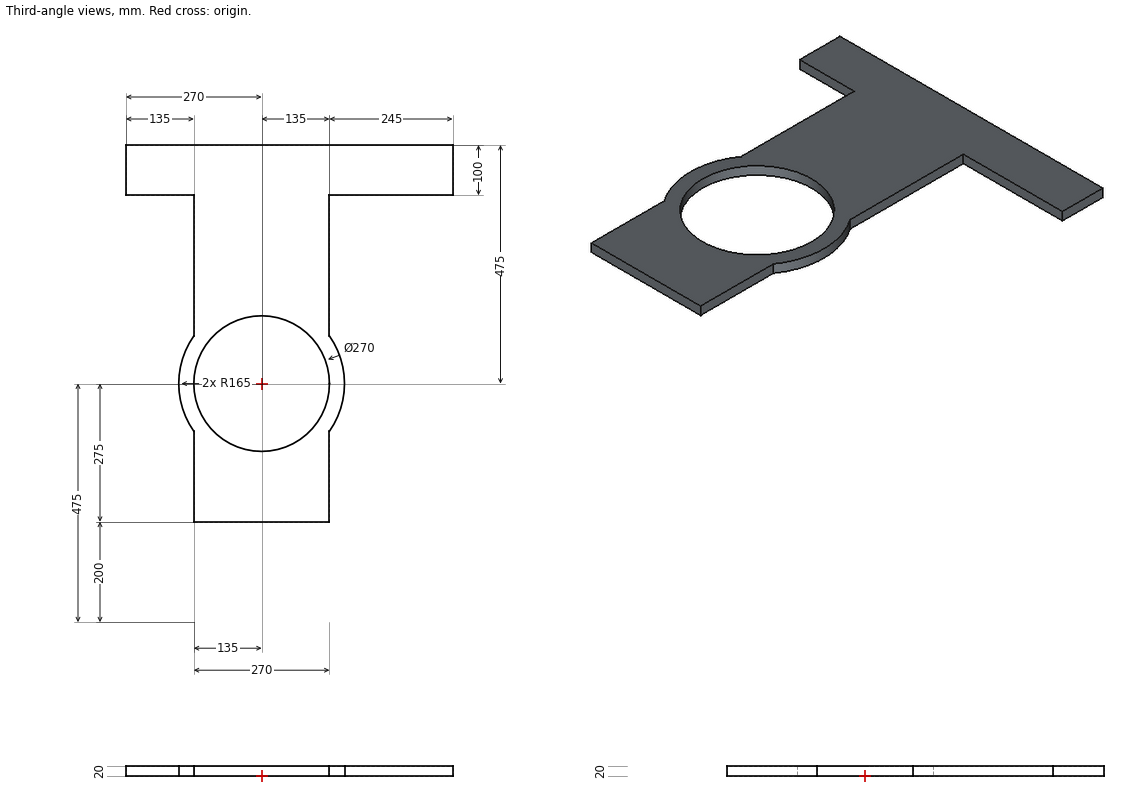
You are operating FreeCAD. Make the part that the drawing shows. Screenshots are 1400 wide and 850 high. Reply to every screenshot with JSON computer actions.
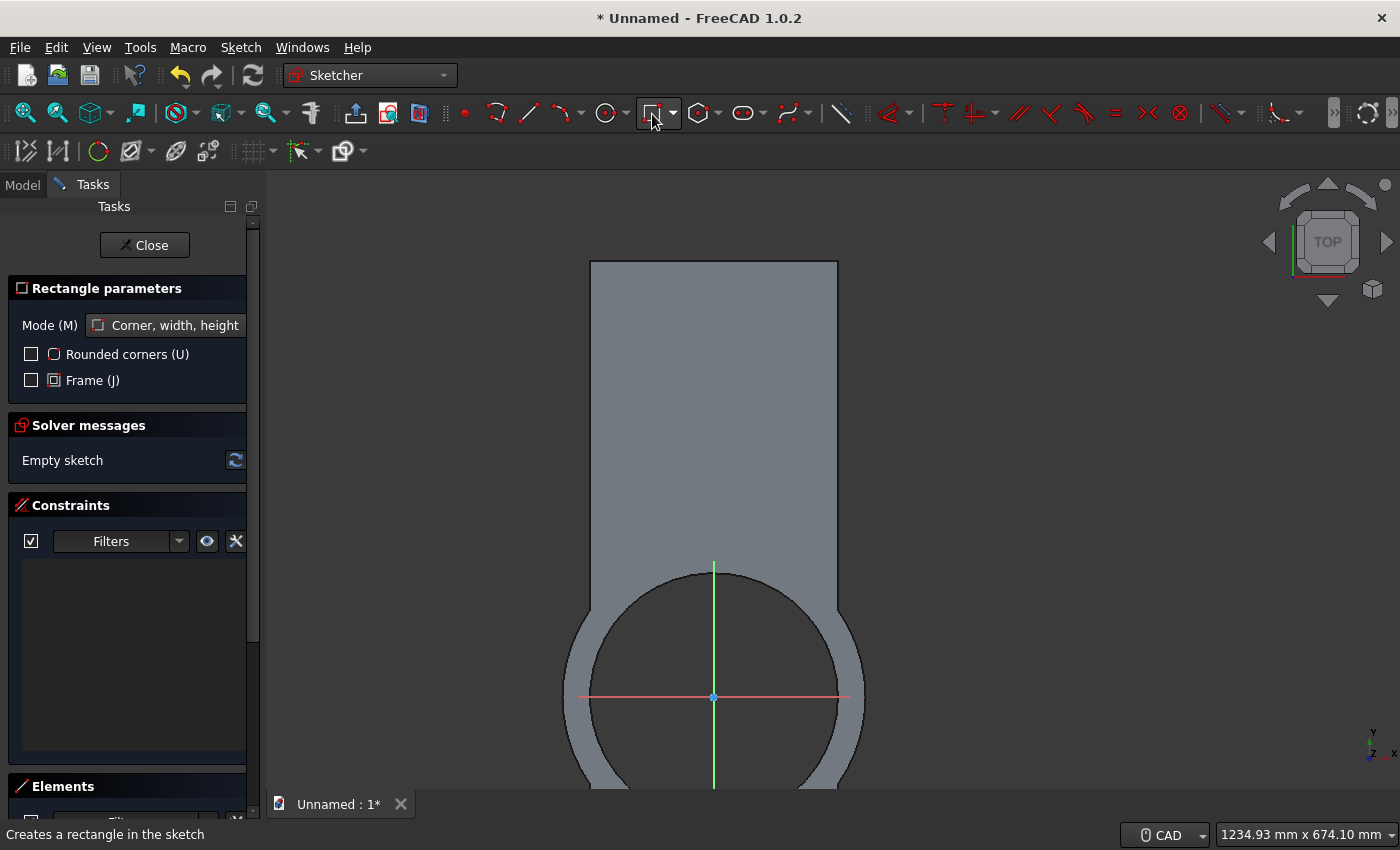
{"action": "left_click", "coordinate": [838, 261]}
{"action": "left_click", "coordinate": [1063, 353]}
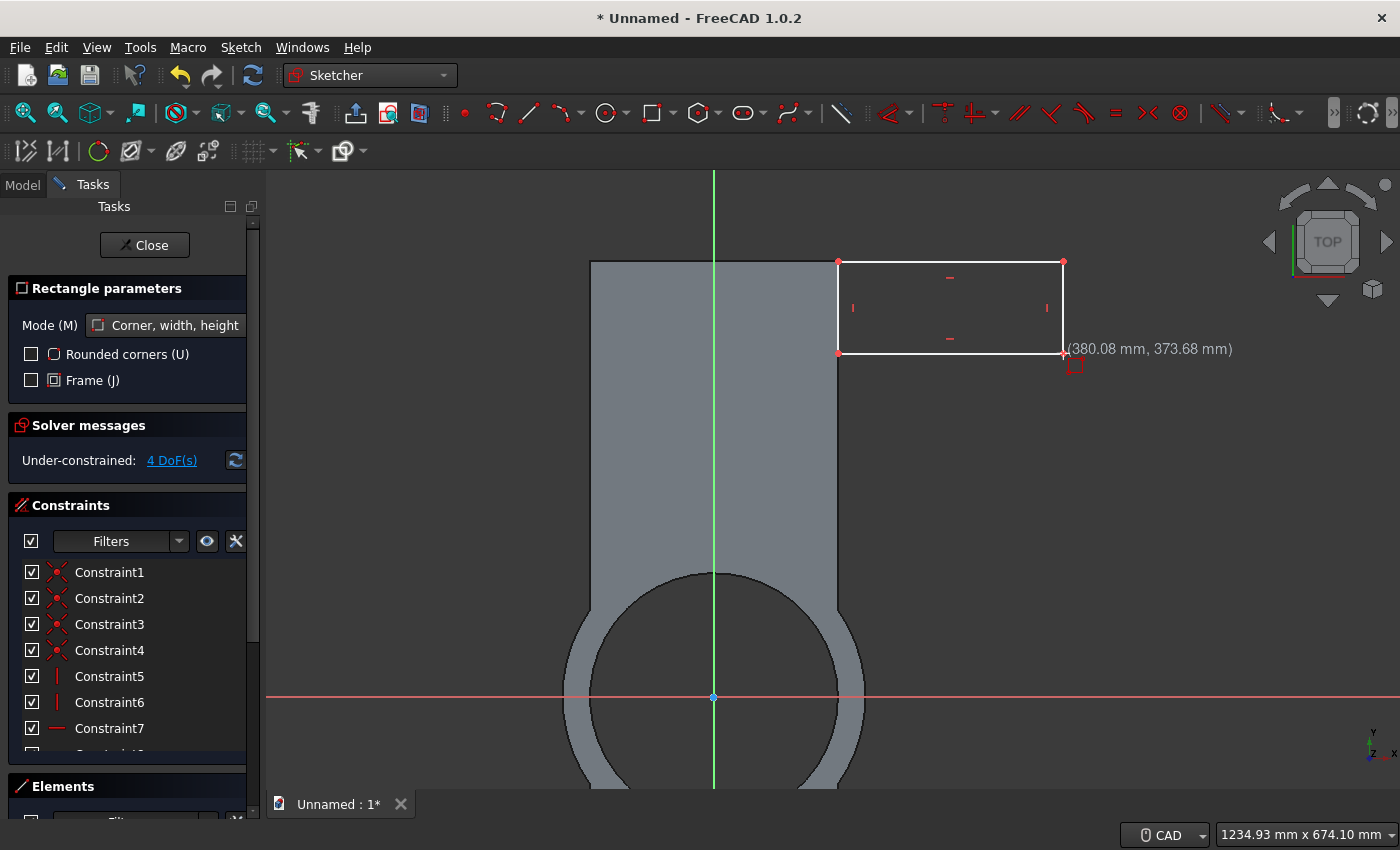
{"action": "left_click", "coordinate": [466, 261]}
{"action": "left_click", "coordinate": [590, 353]}
{"action": "key", "text": "Escape"}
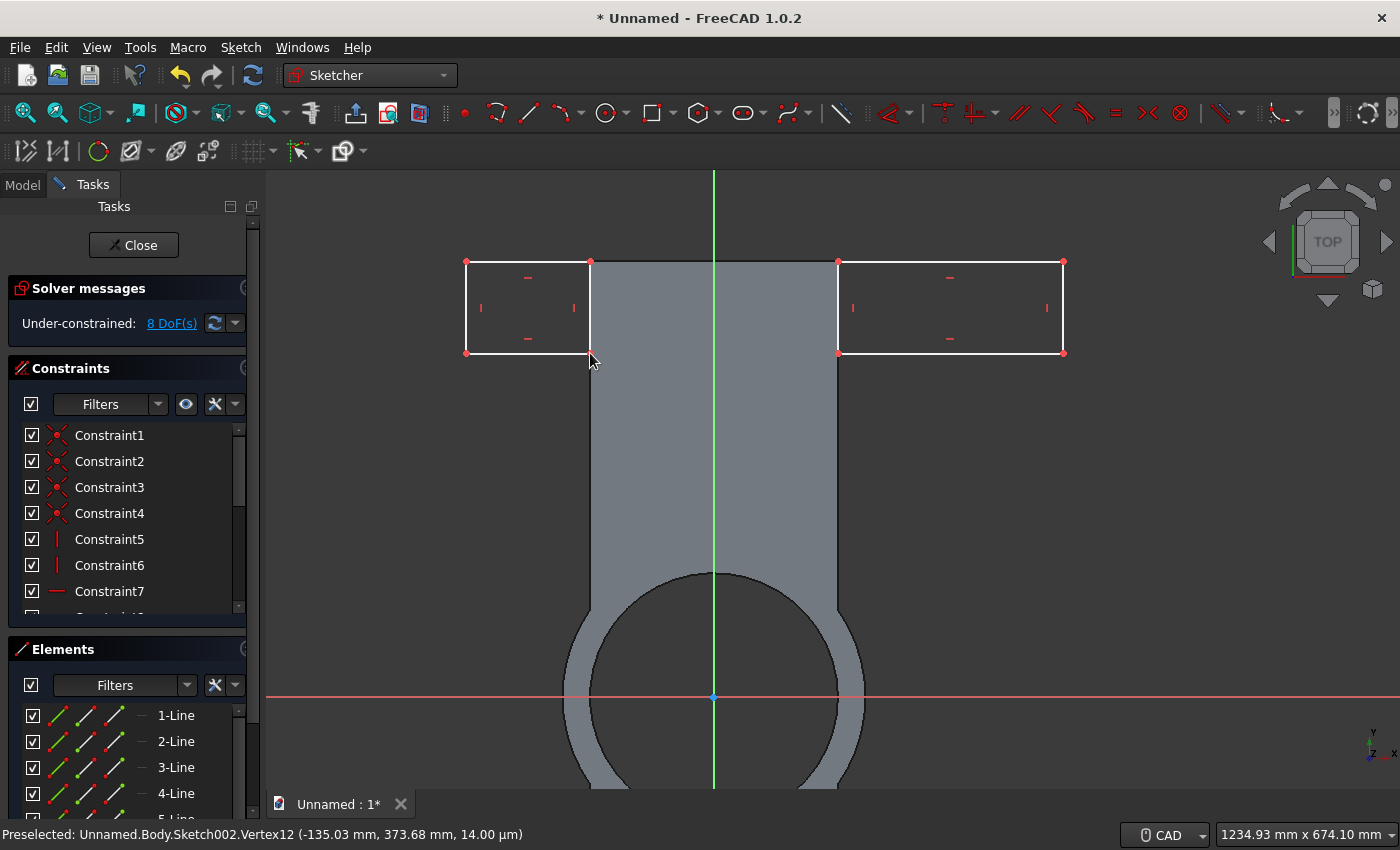
{"action": "left_click", "coordinate": [888, 114]}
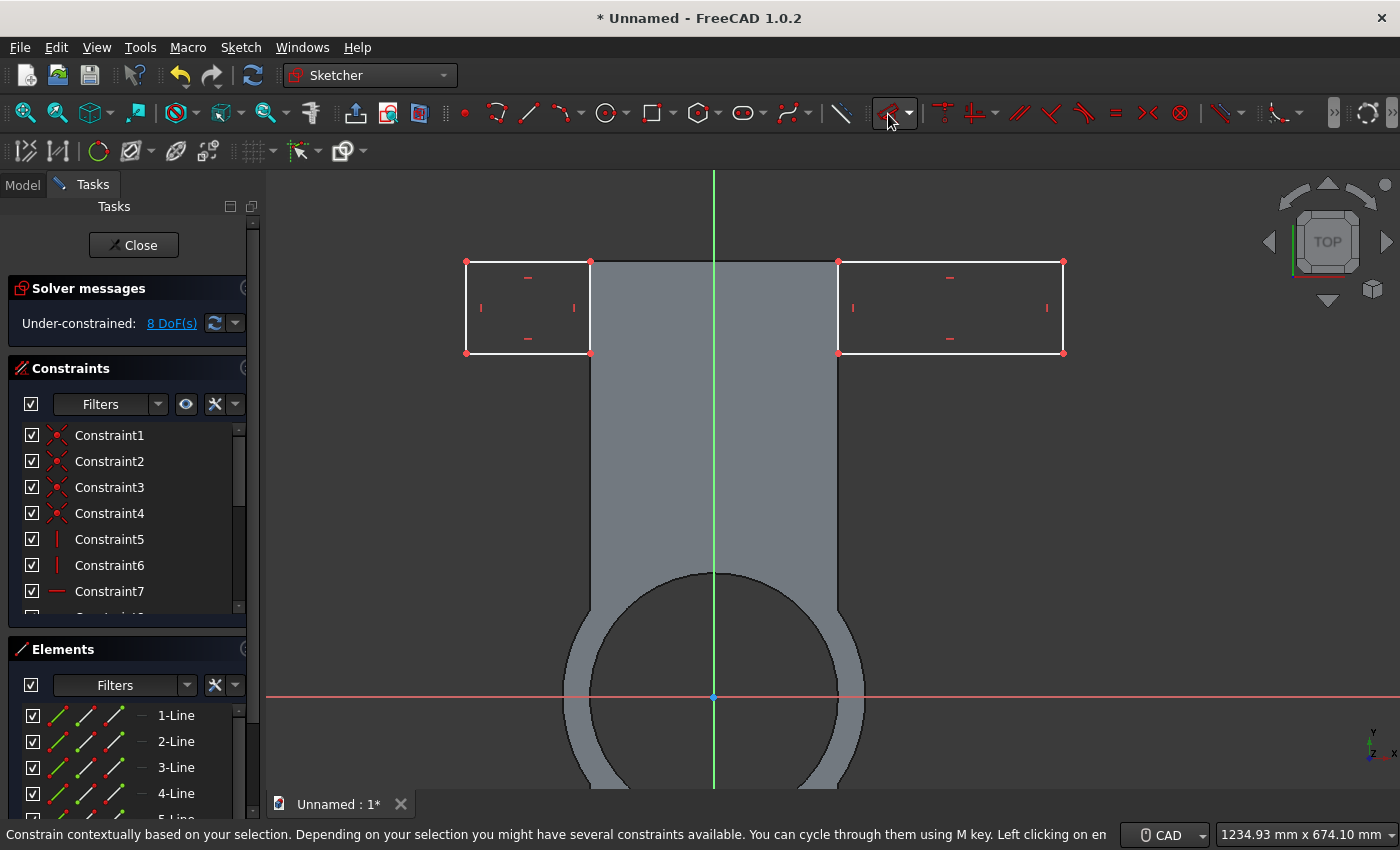
{"action": "left_click", "coordinate": [838, 290]}
{"action": "left_click", "coordinate": [872, 308]}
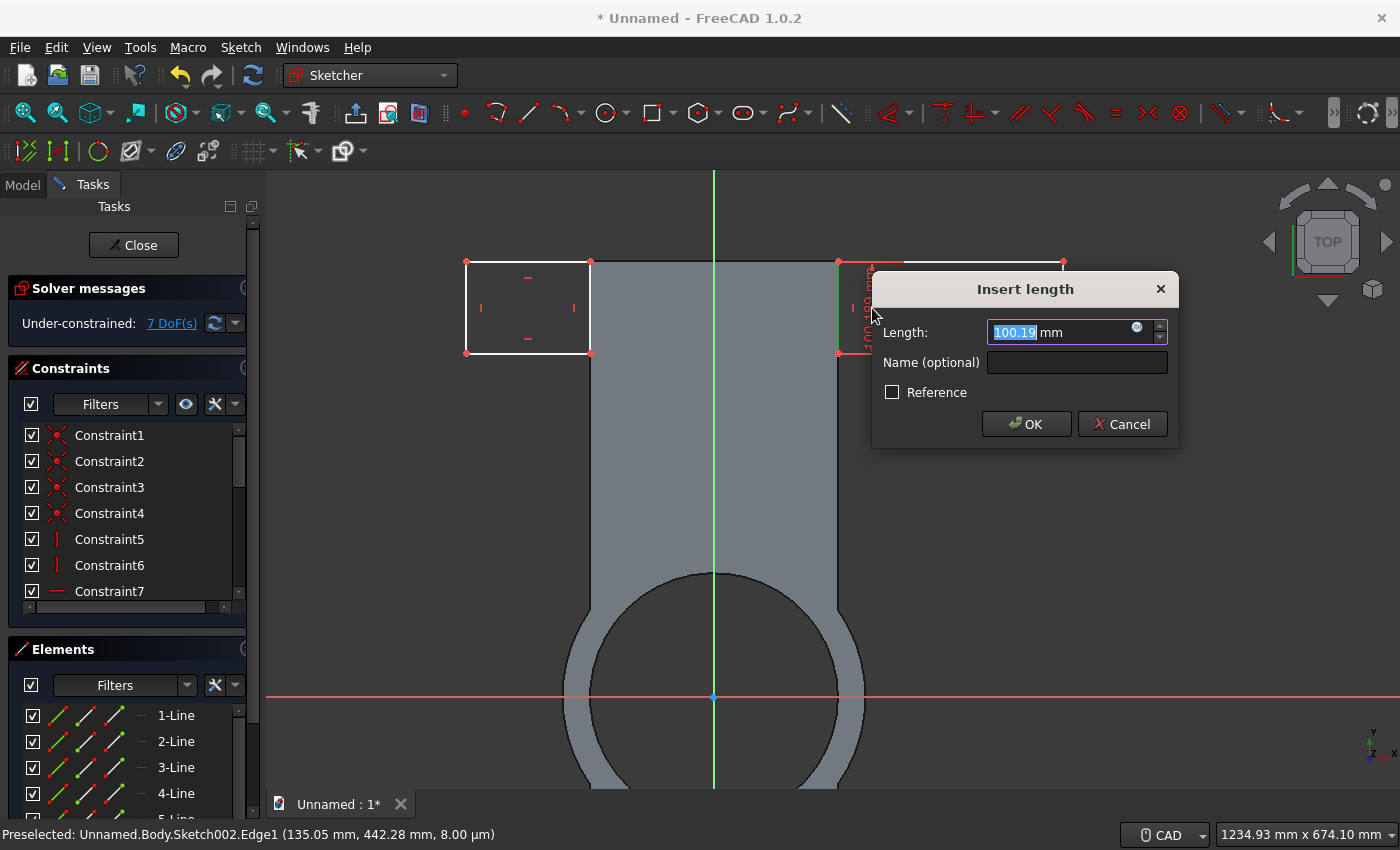
{"action": "type", "text": "100"}
{"action": "key", "text": "Return"}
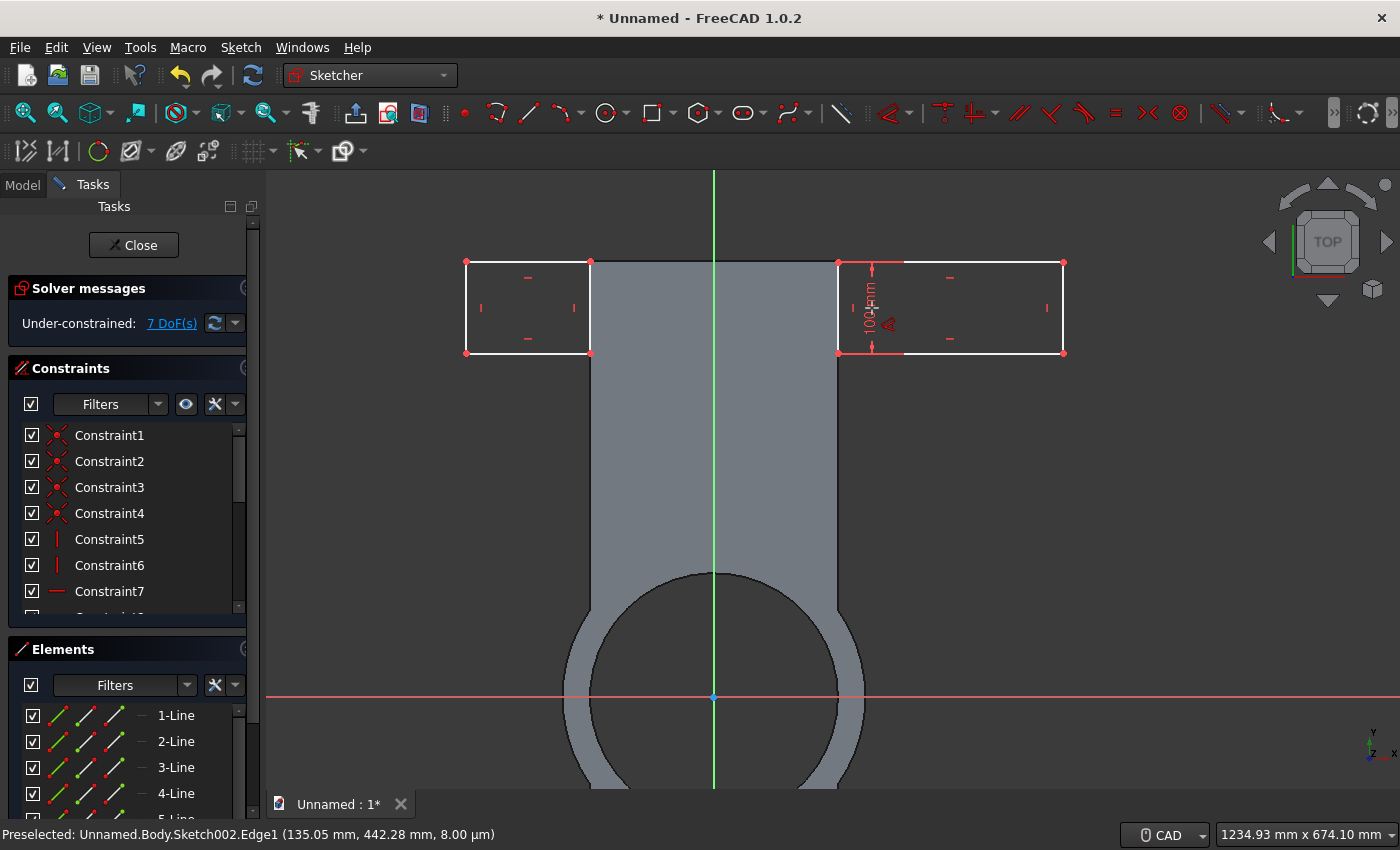
{"action": "left_click", "coordinate": [906, 354]}
{"action": "left_click", "coordinate": [950, 320]}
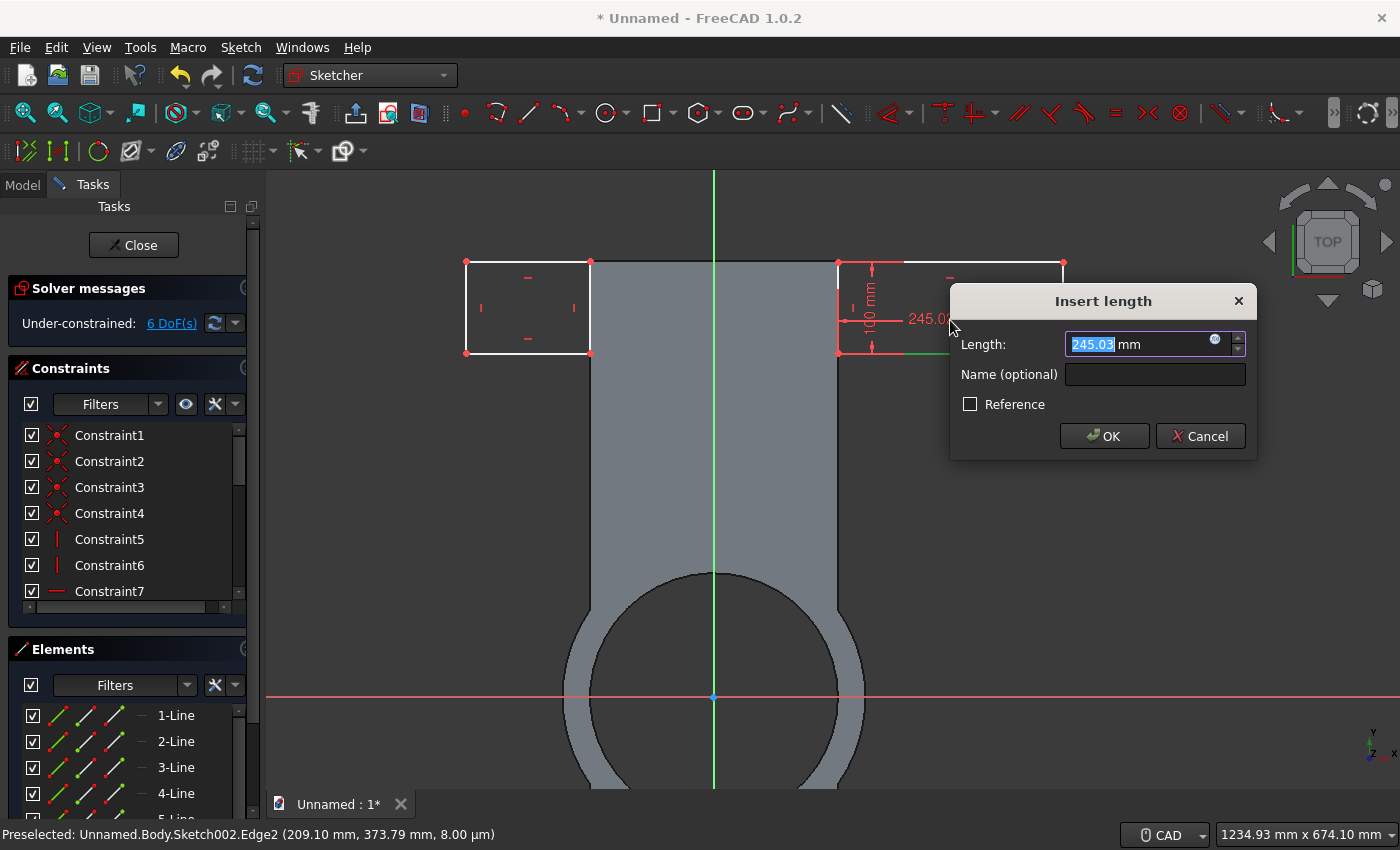
{"action": "type", "text": "245"}
{"action": "key", "text": "Return"}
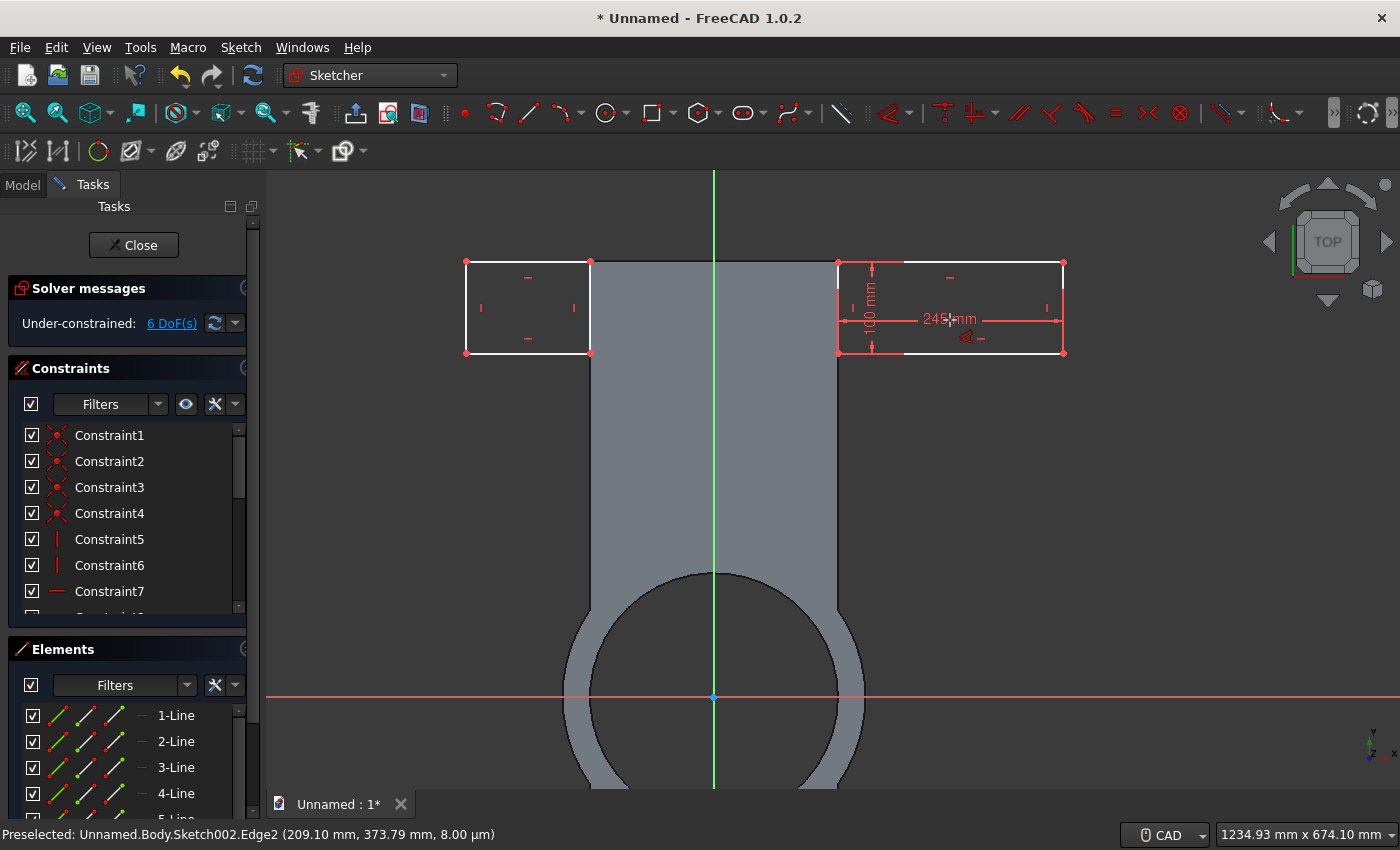
{"action": "left_click", "coordinate": [466, 290]}
{"action": "left_click", "coordinate": [432, 308]}